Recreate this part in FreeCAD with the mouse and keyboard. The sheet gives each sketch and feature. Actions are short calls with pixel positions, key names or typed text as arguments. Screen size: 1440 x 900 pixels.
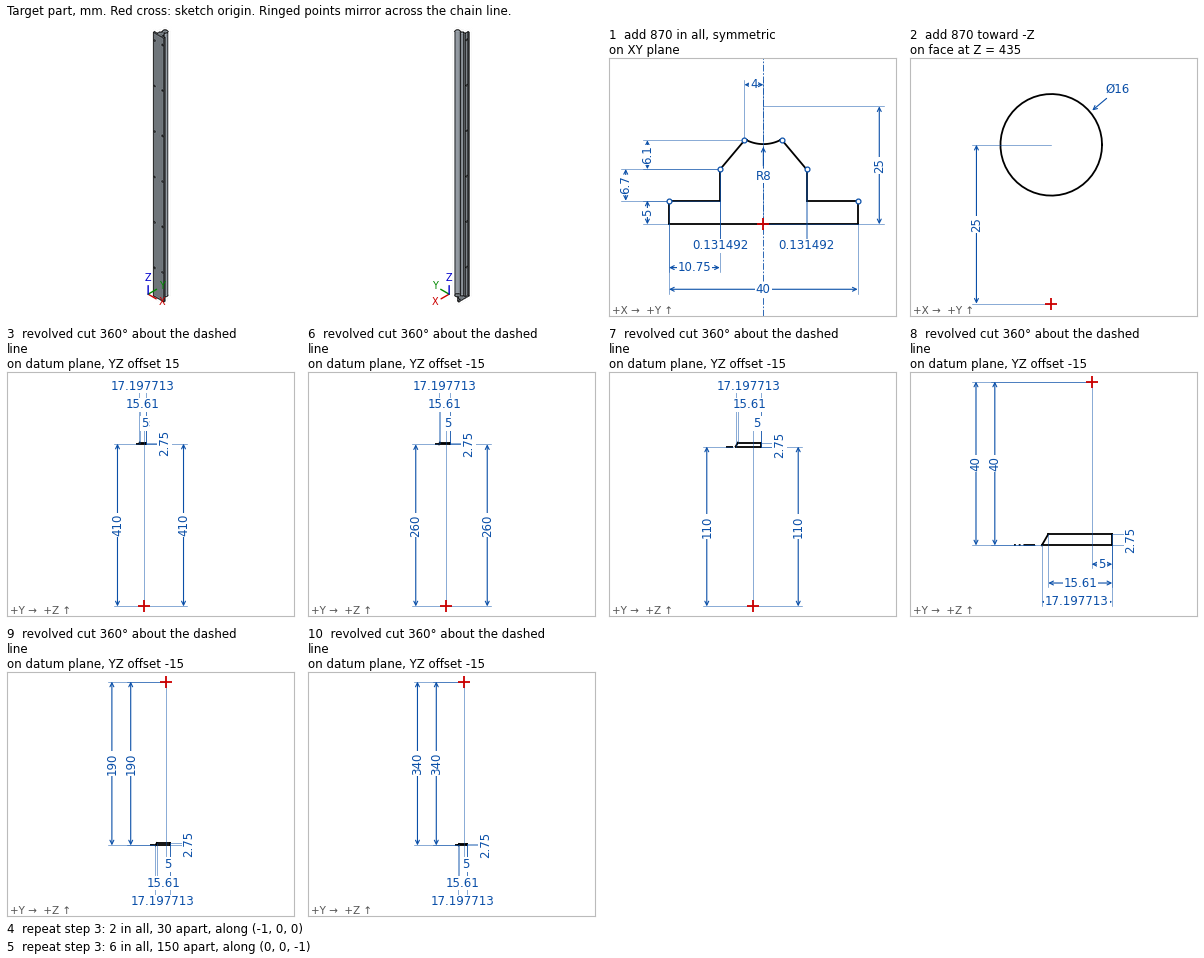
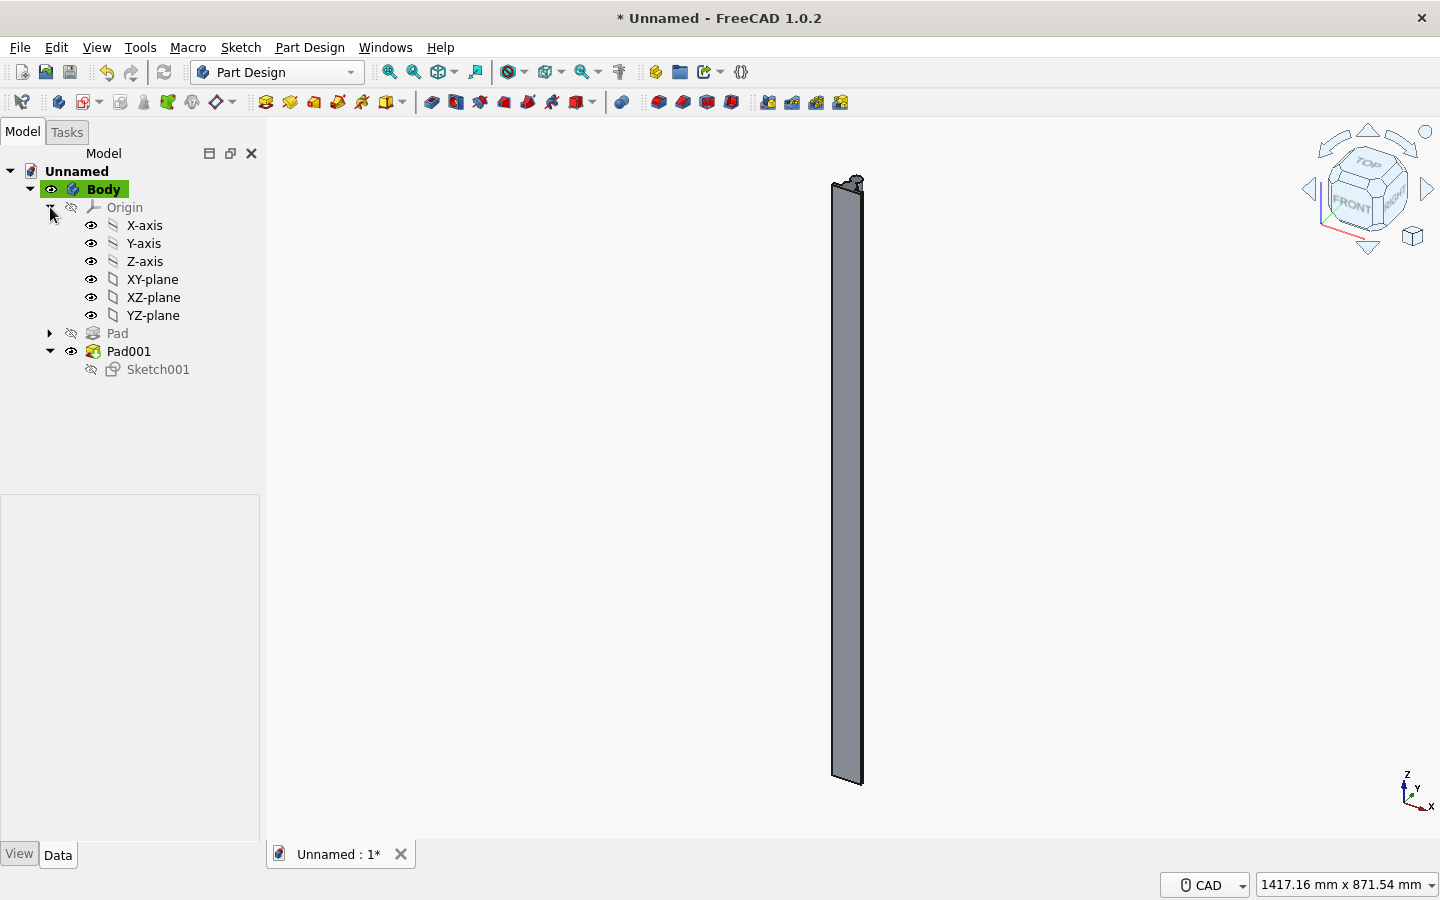
click(136, 315)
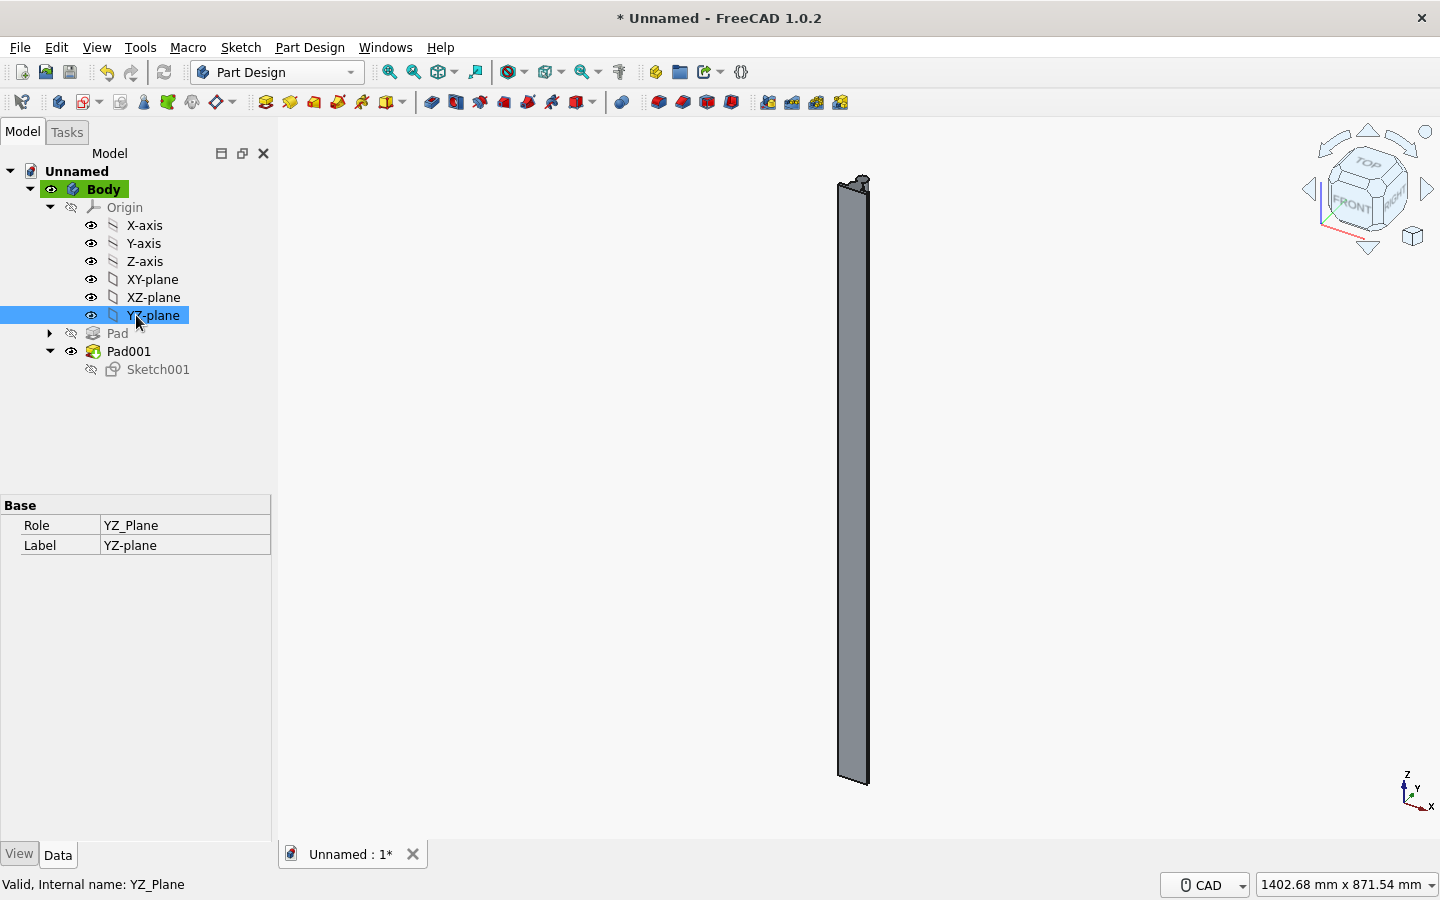
click(216, 102)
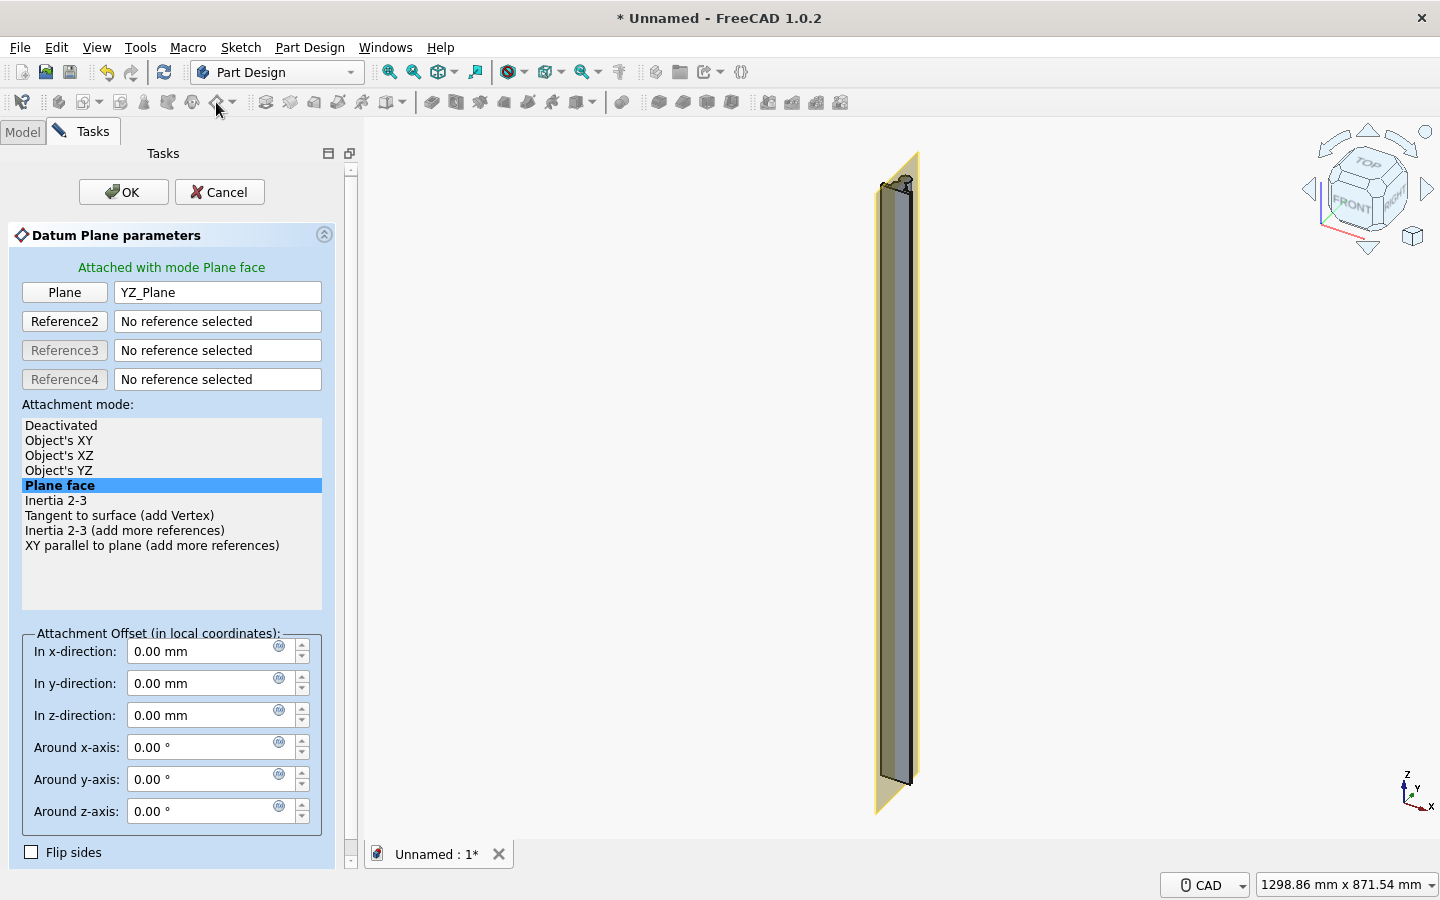
triple_click(210, 715)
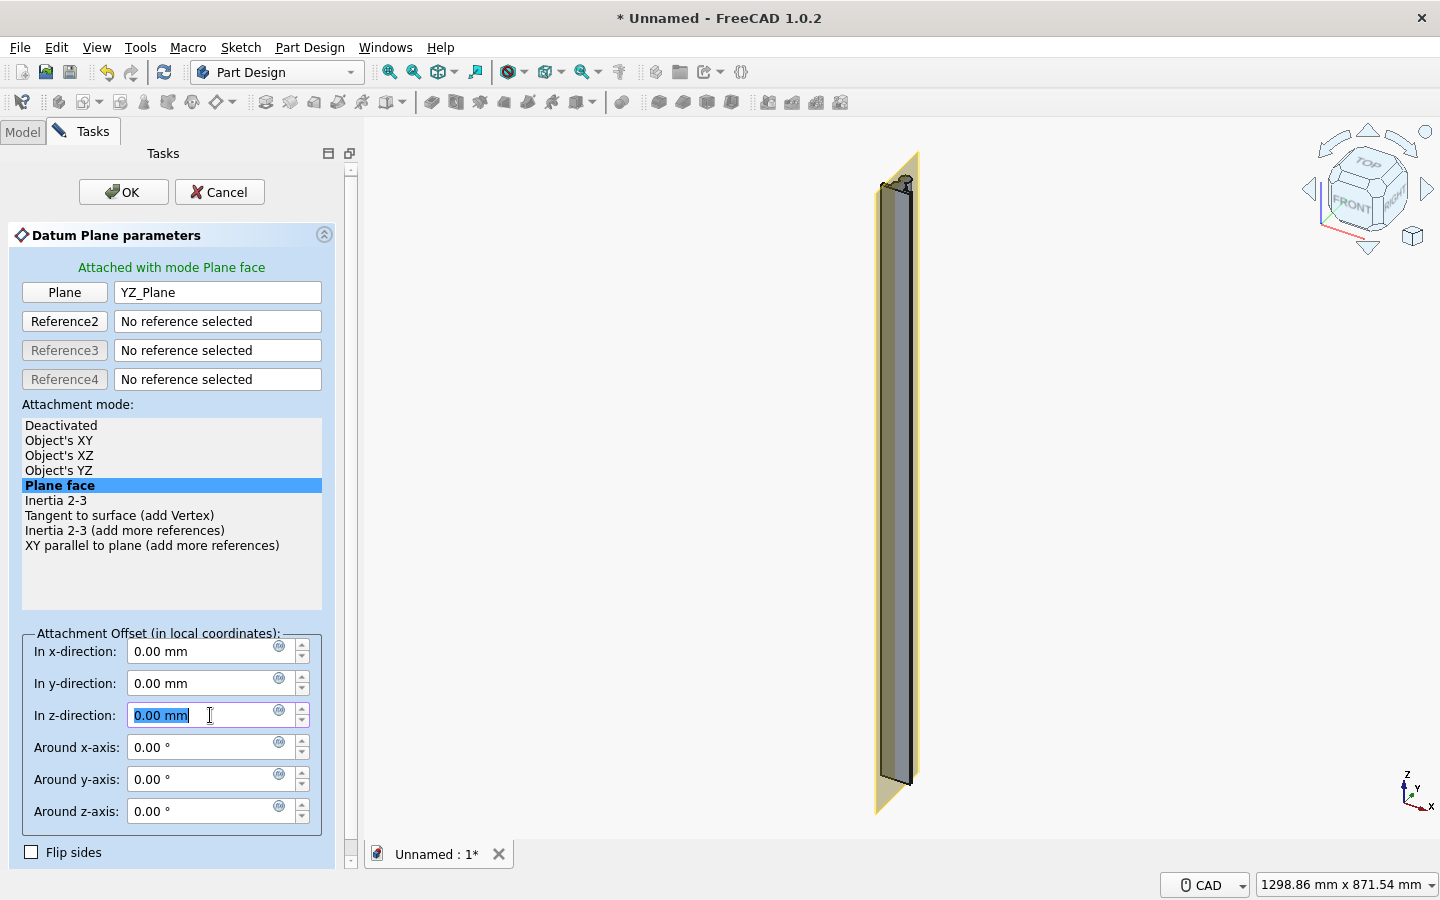
text(15)
key(Tab)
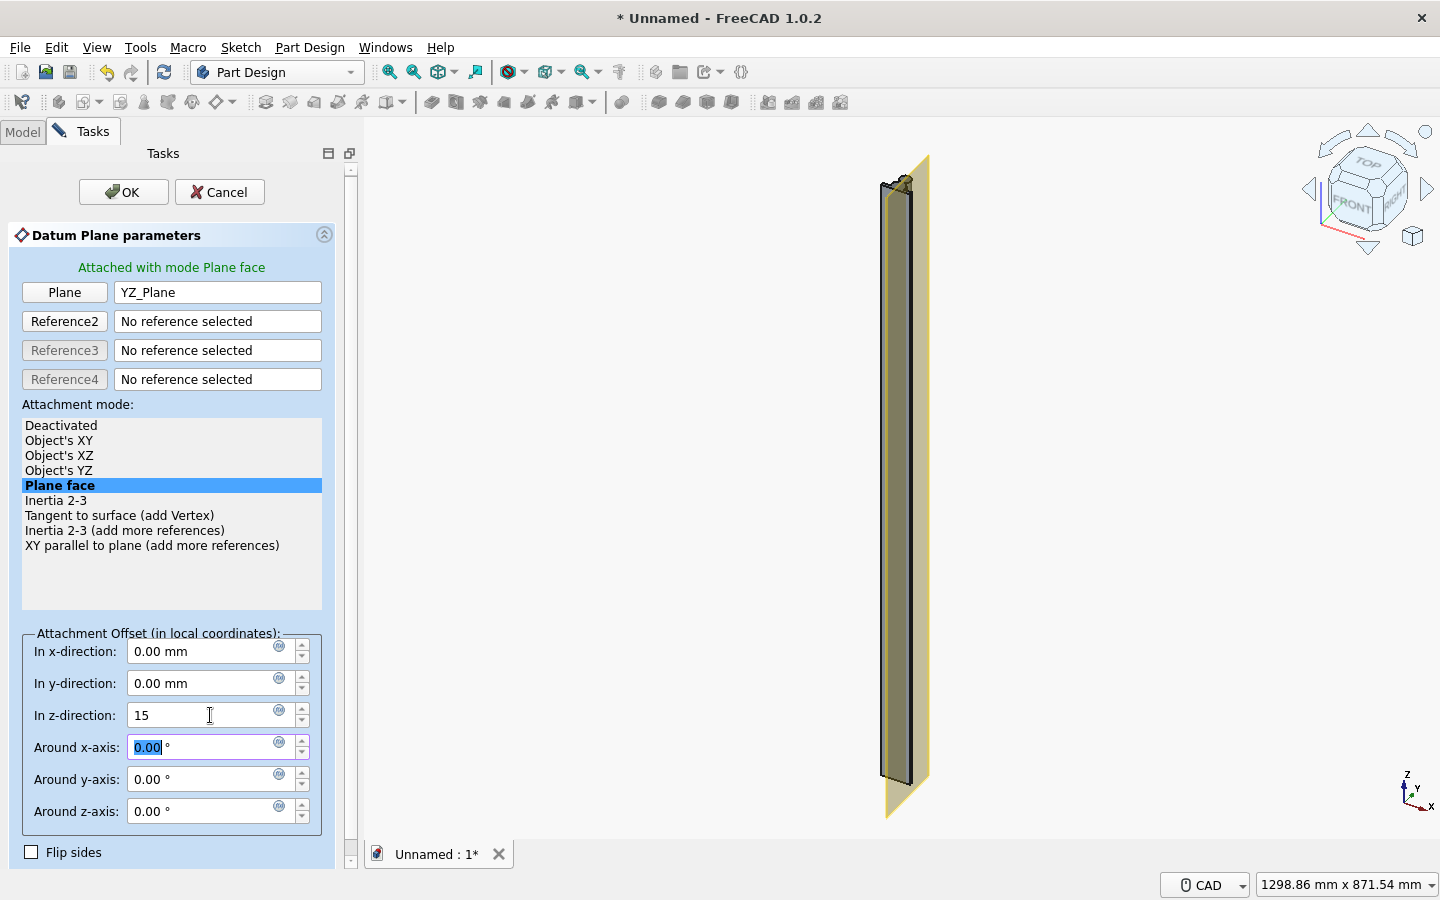
click(124, 192)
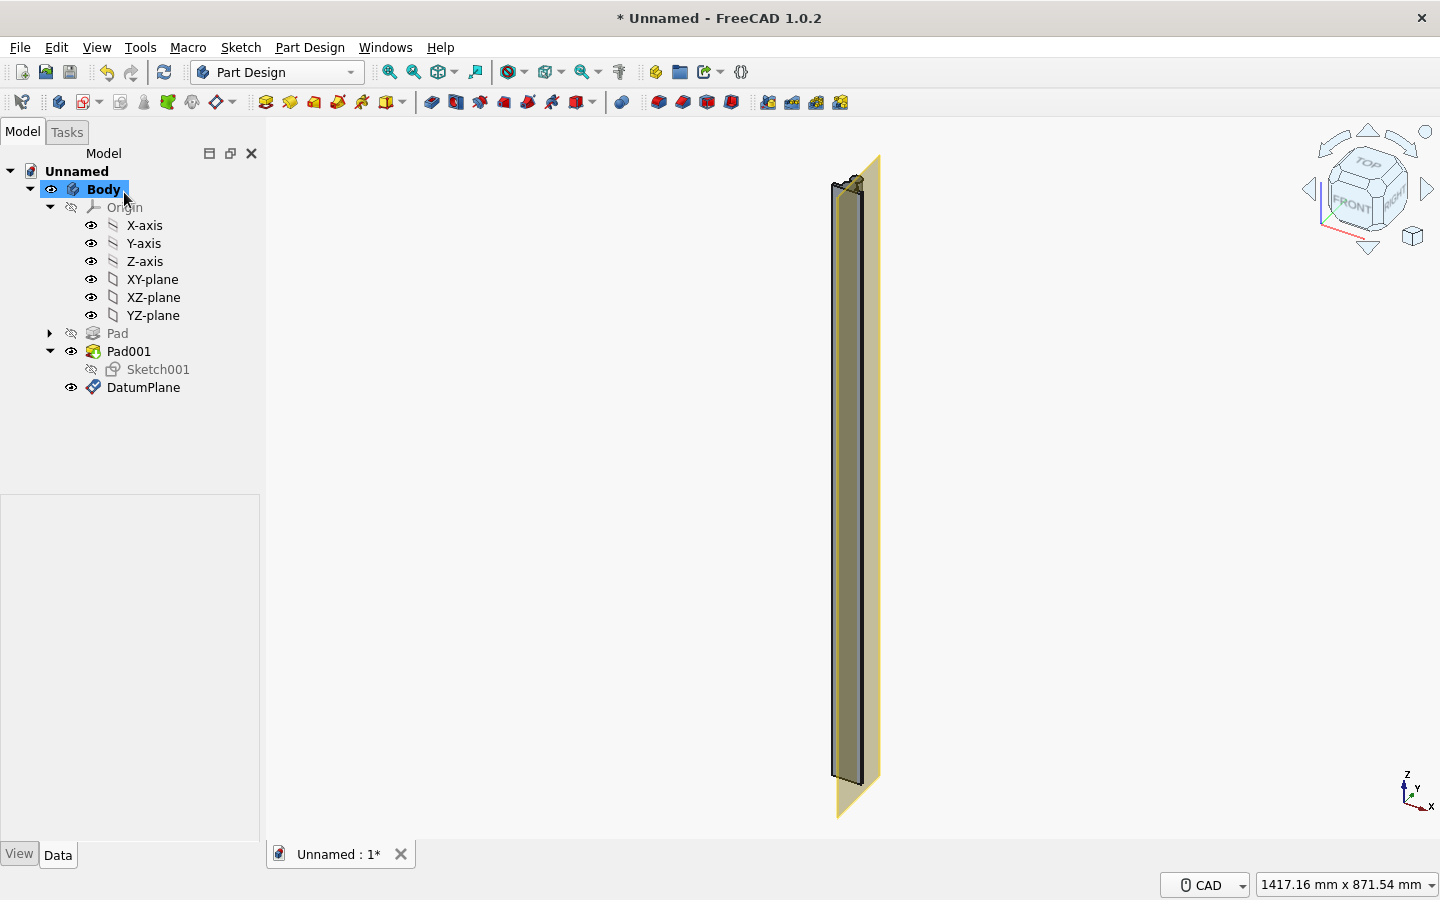
click(116, 387)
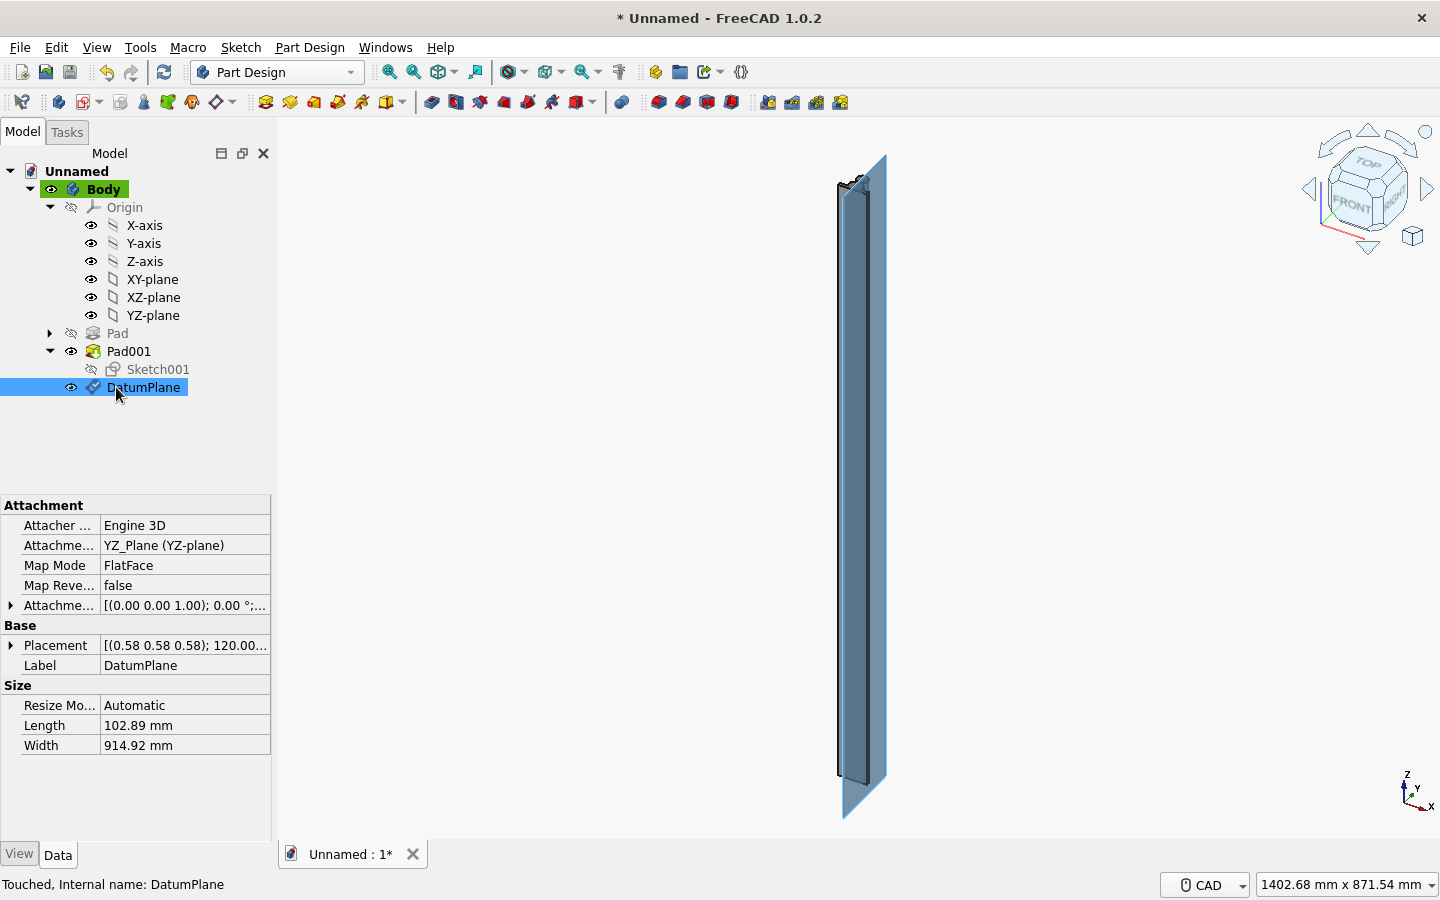
click(84, 102)